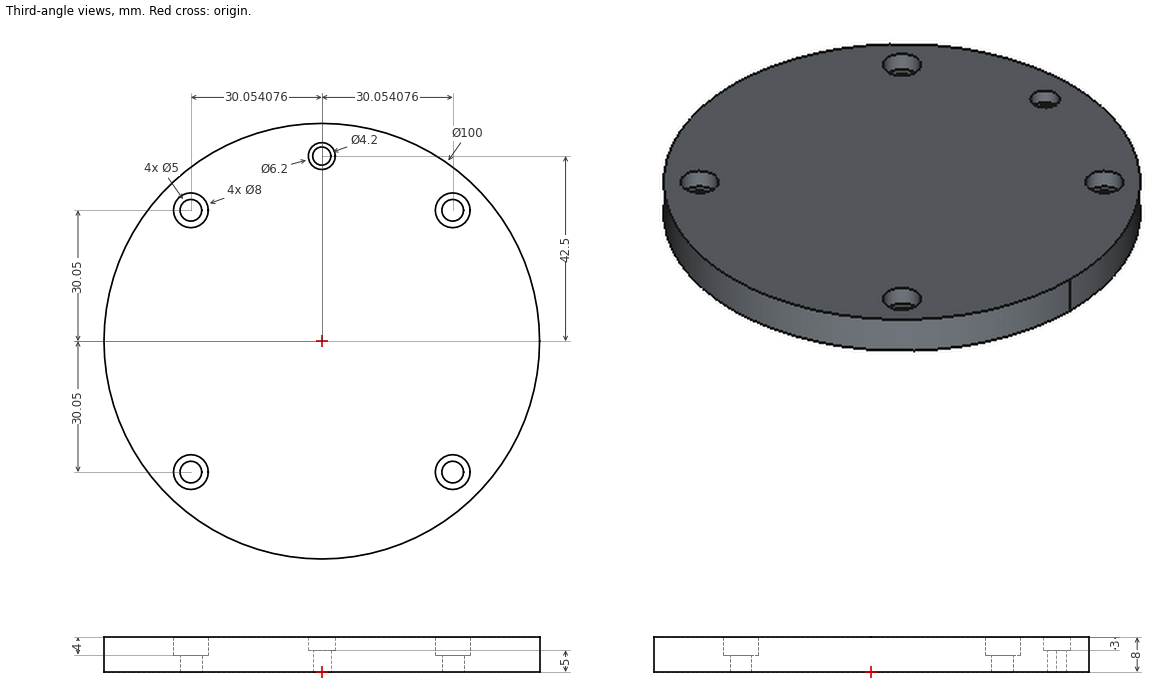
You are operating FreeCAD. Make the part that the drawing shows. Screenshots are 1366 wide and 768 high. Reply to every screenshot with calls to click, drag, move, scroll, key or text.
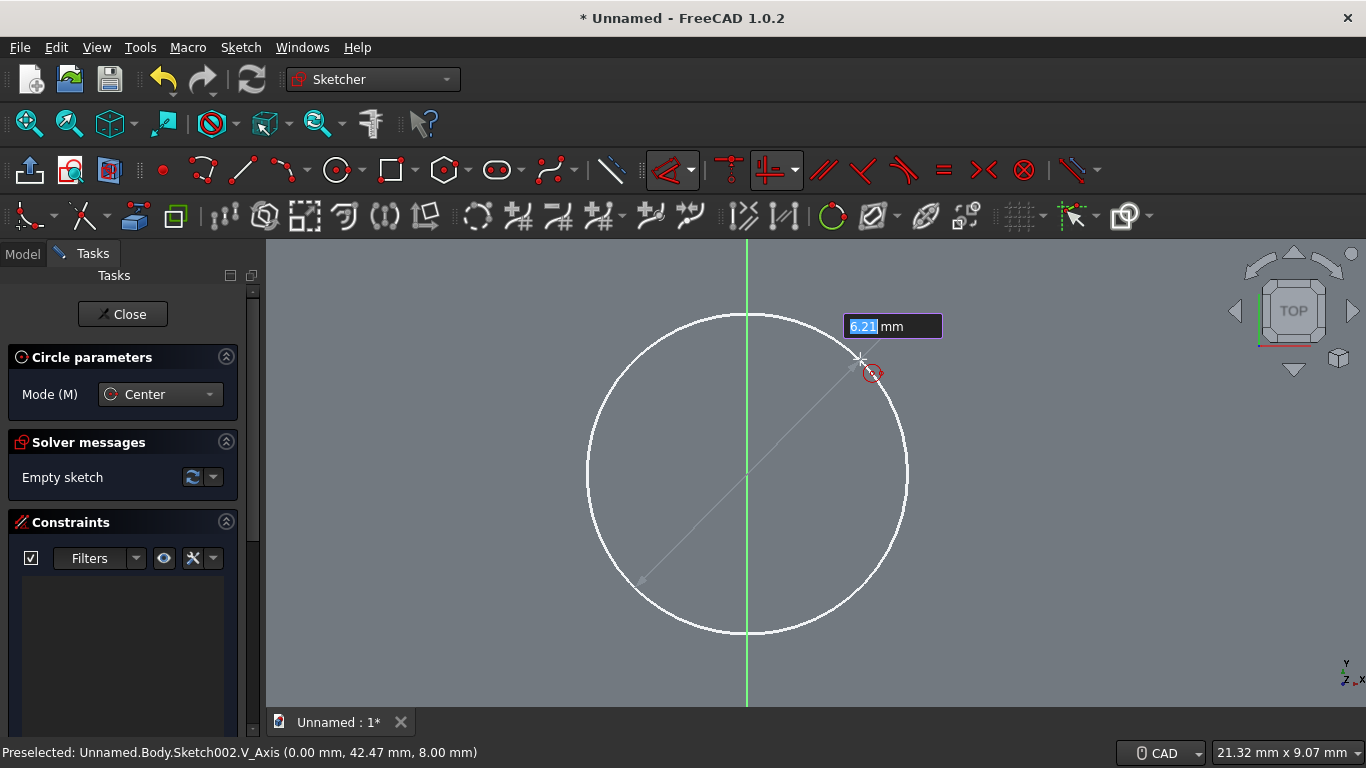
text(6.2)
key(Return)
key(Escape)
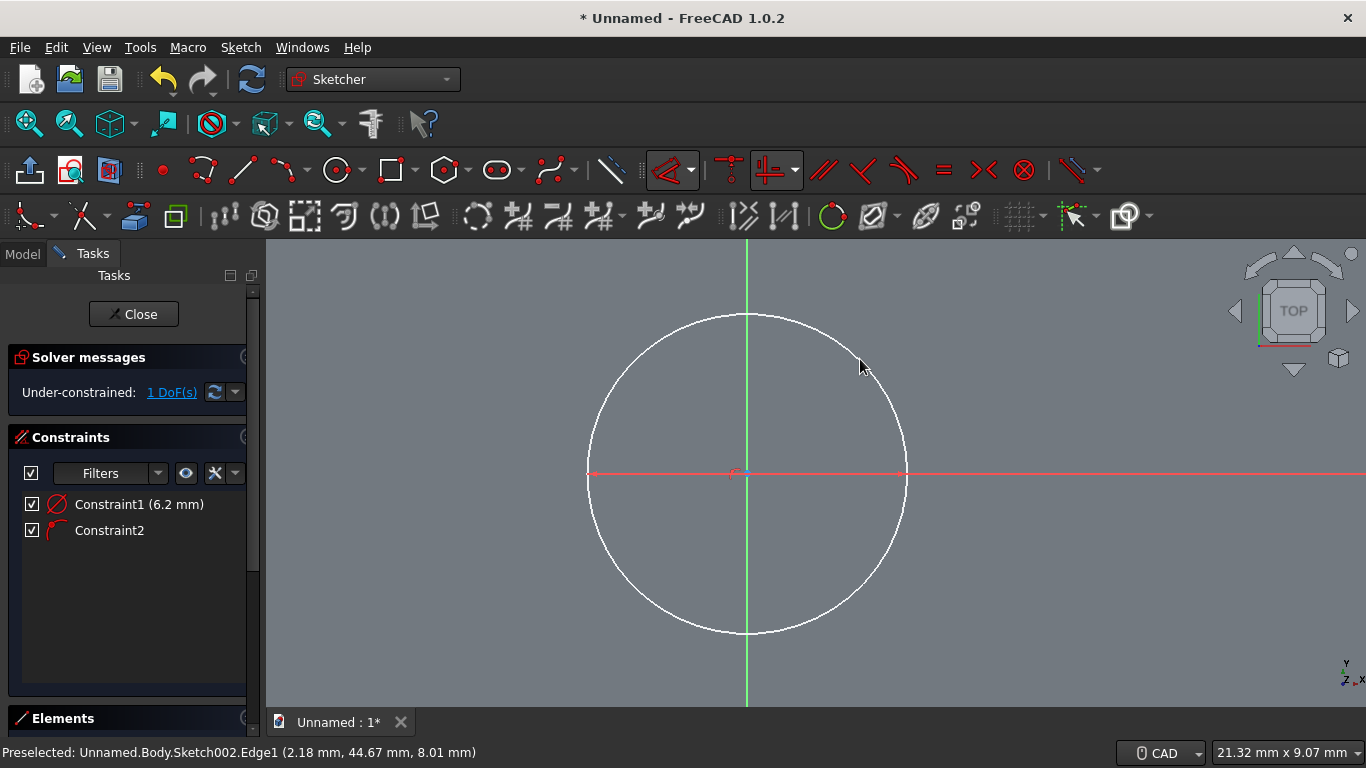
click(747, 474)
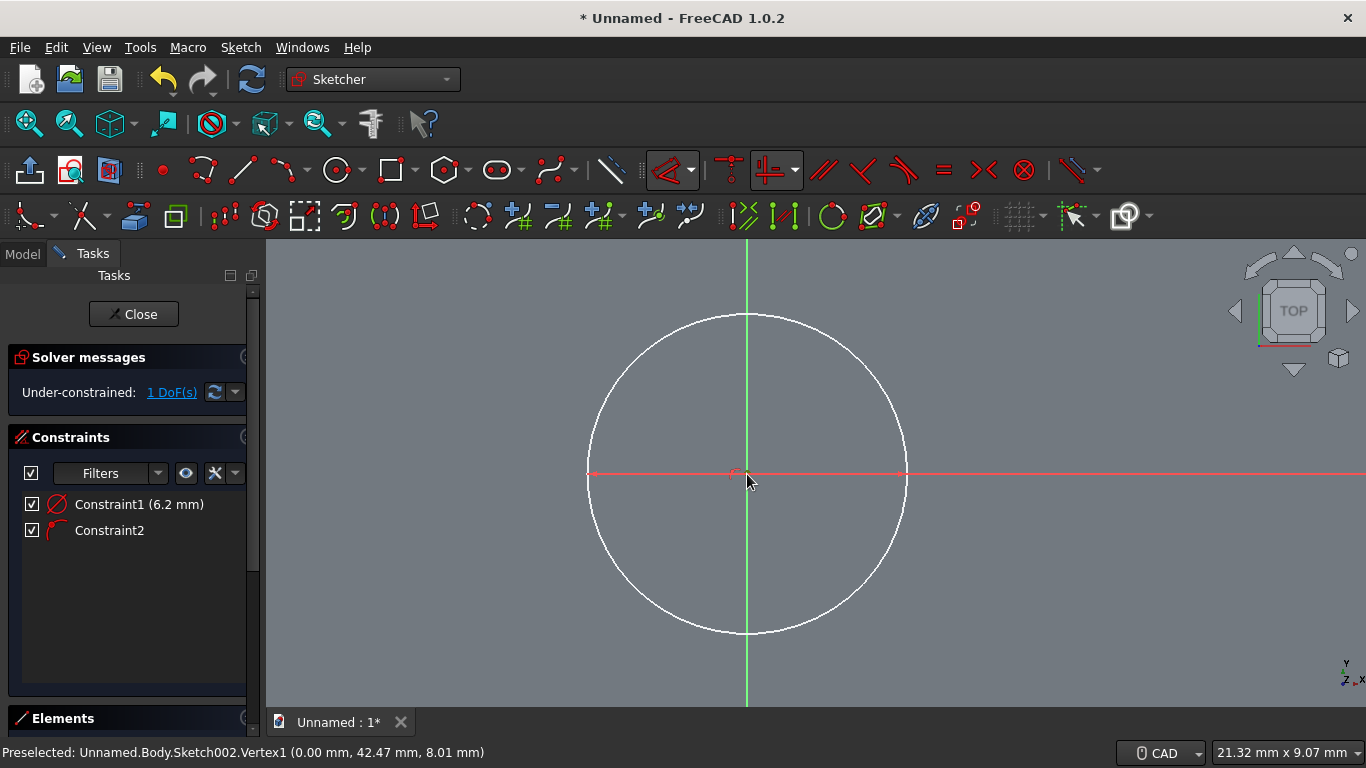
click(694, 170)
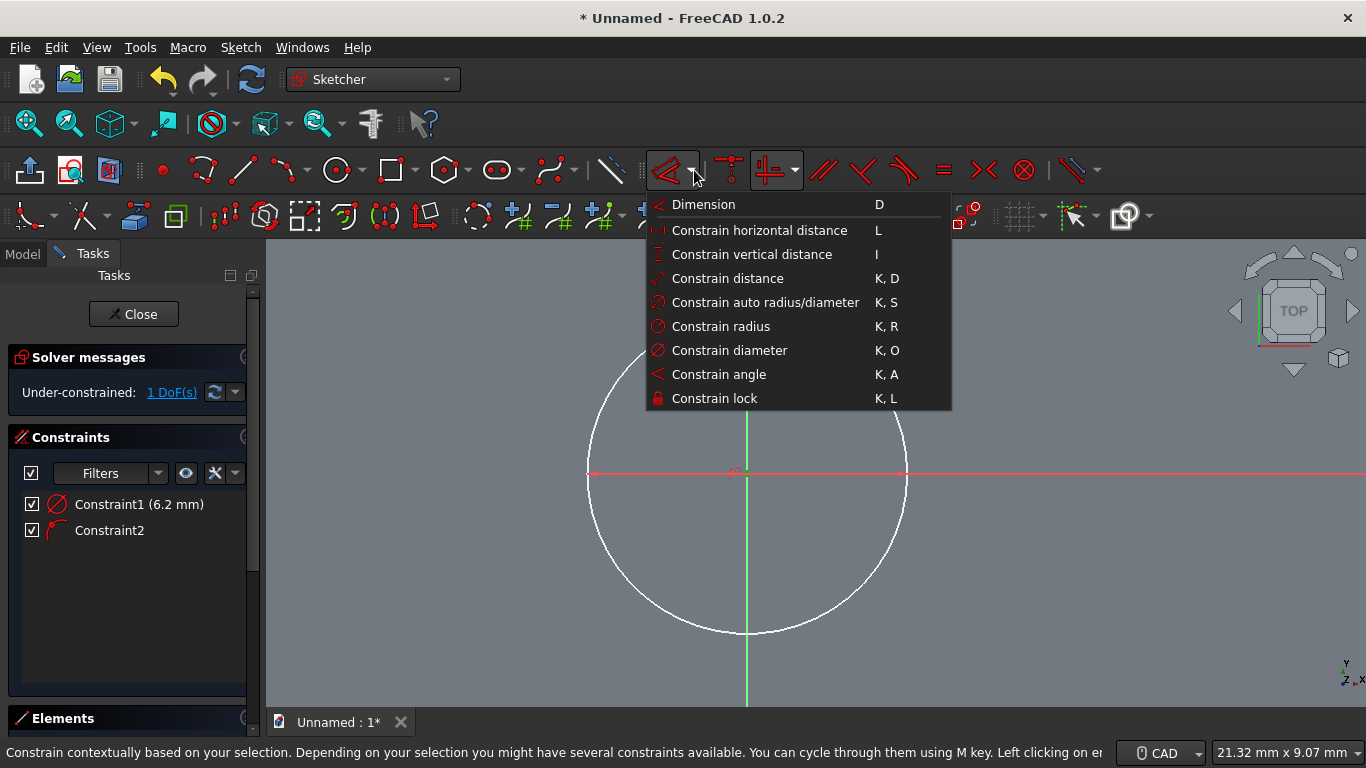
click(799, 254)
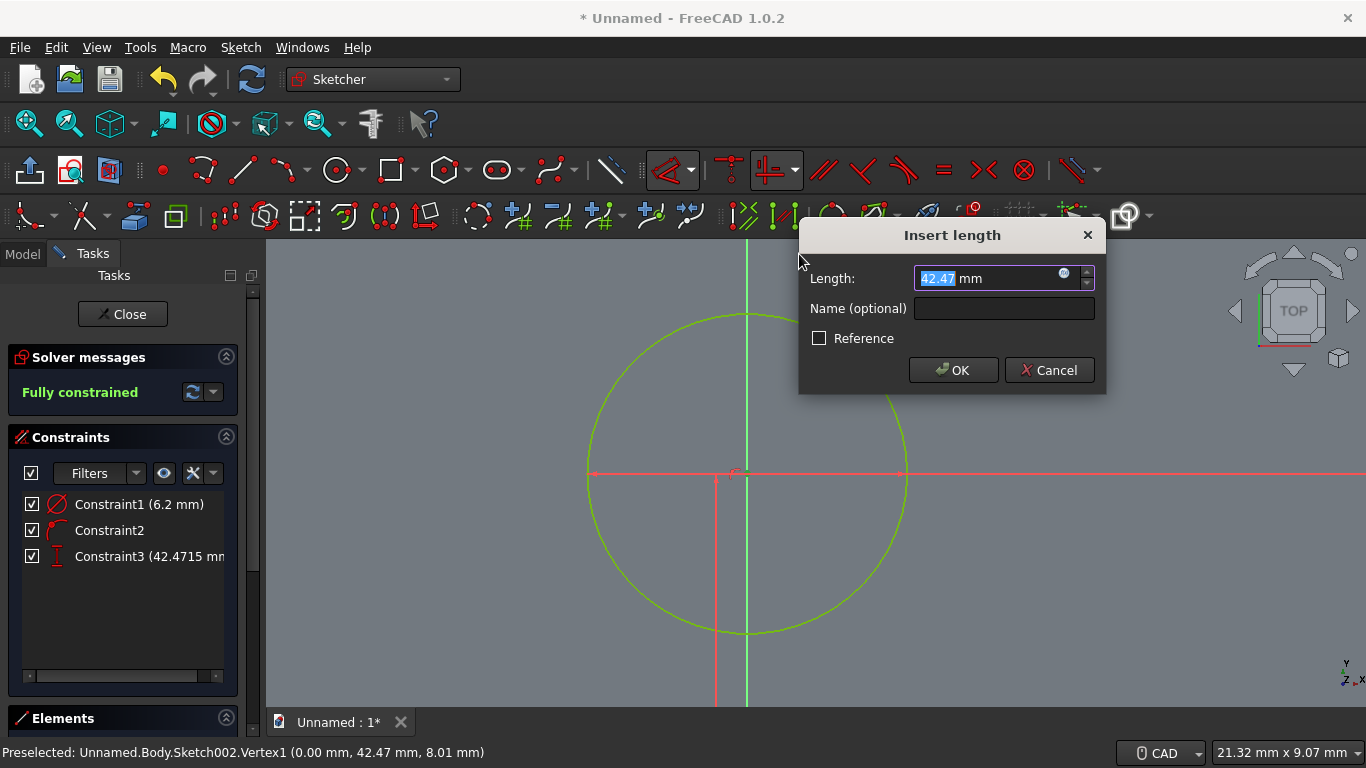
text(42.5)
key(Return)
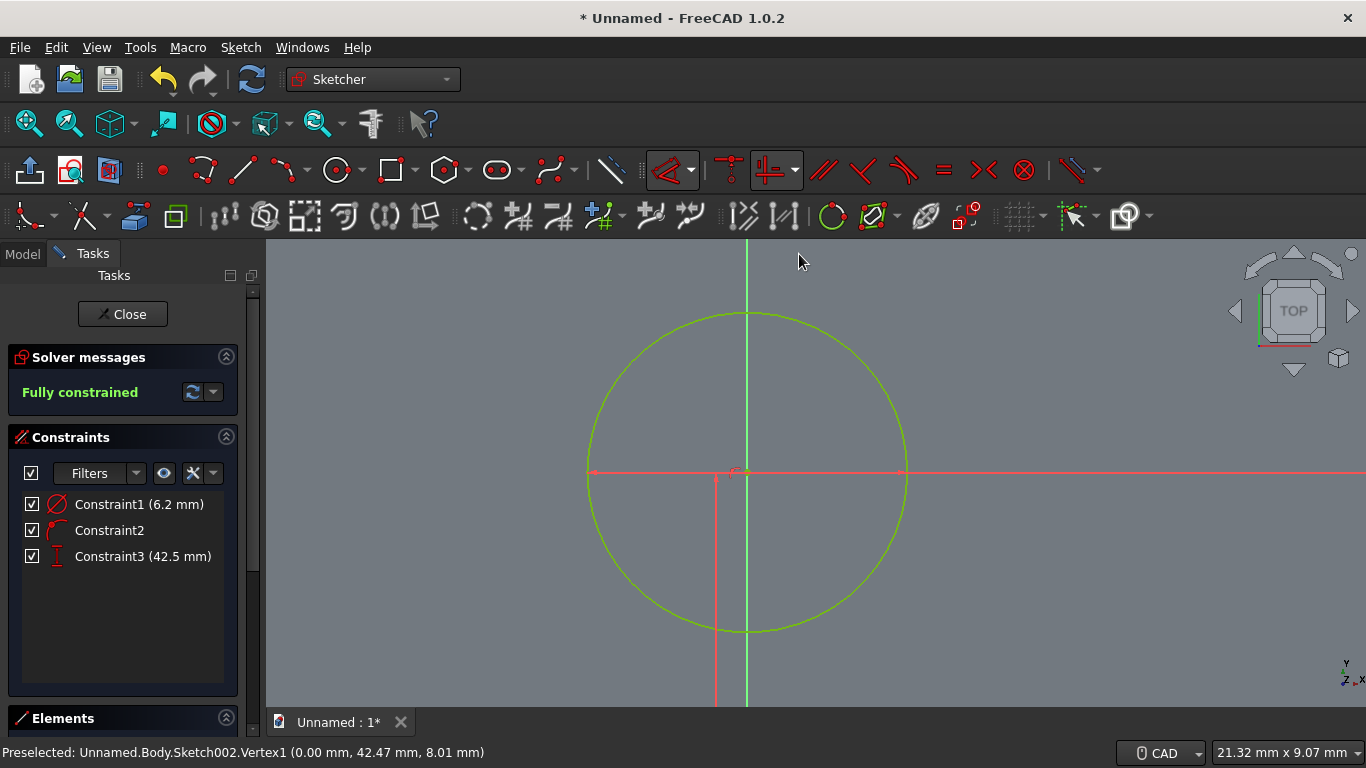
click(123, 314)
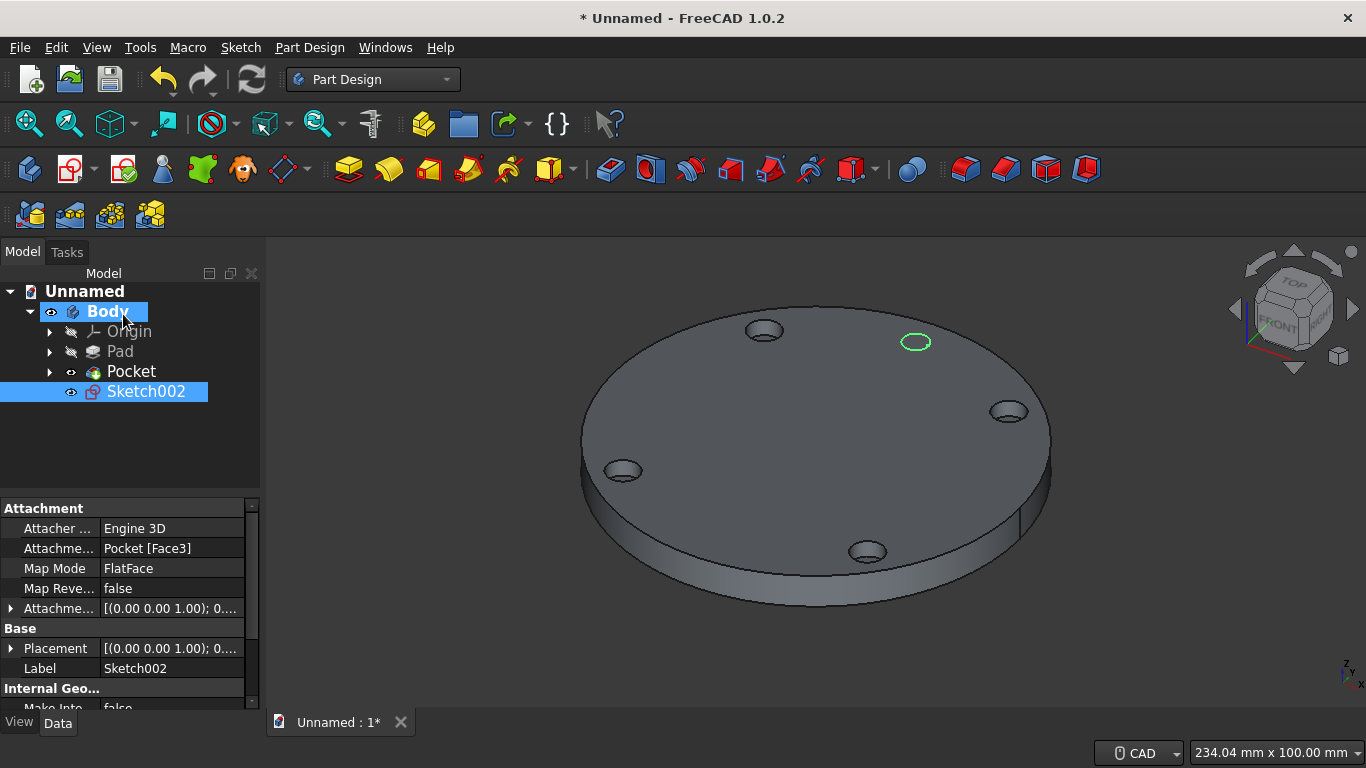
click(612, 170)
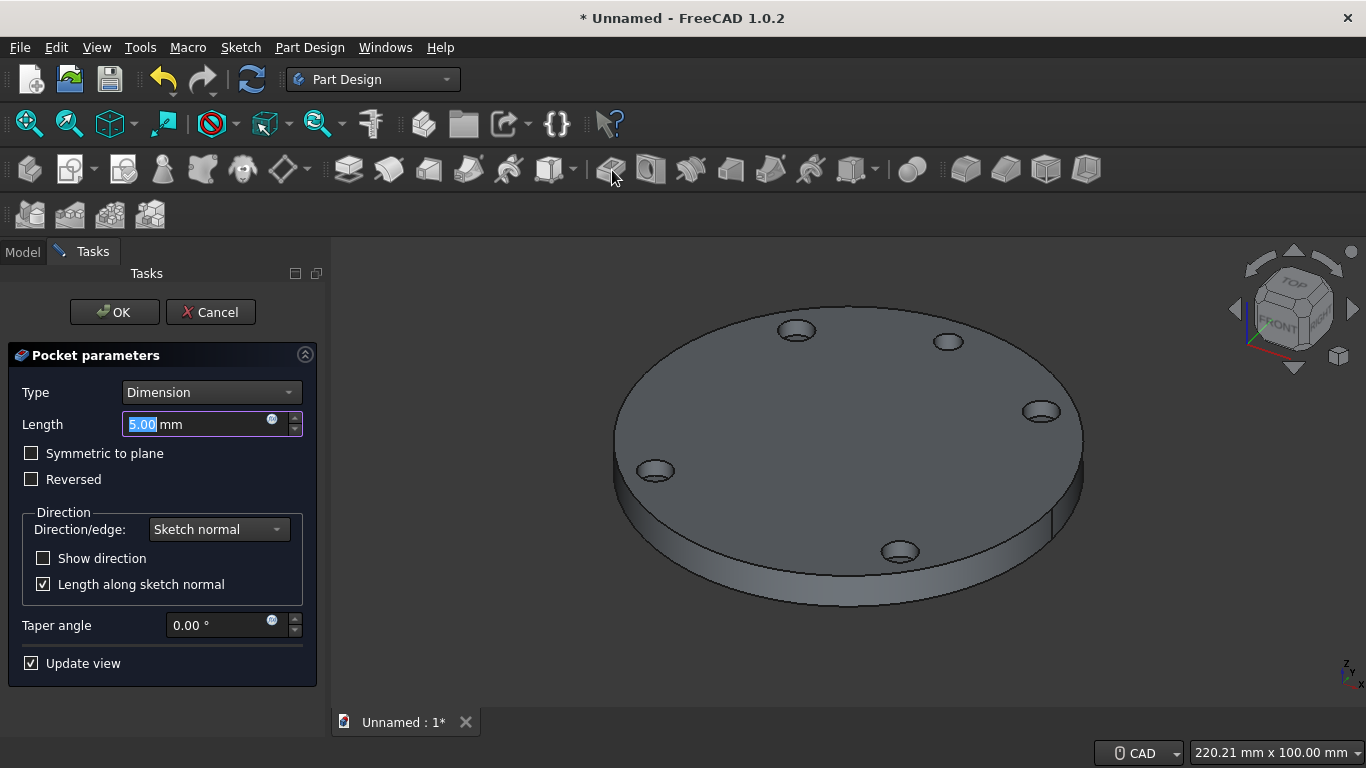
text(3)
key(Tab)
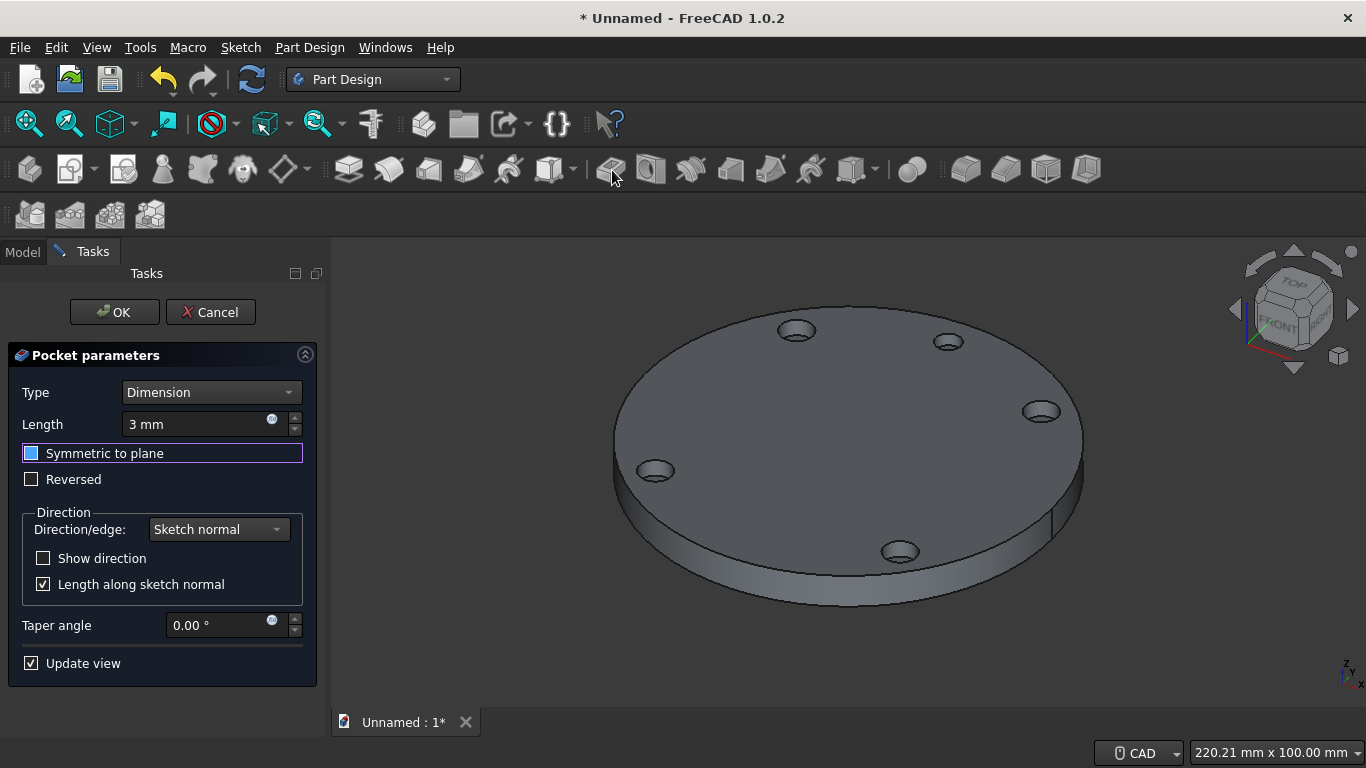
click(115, 312)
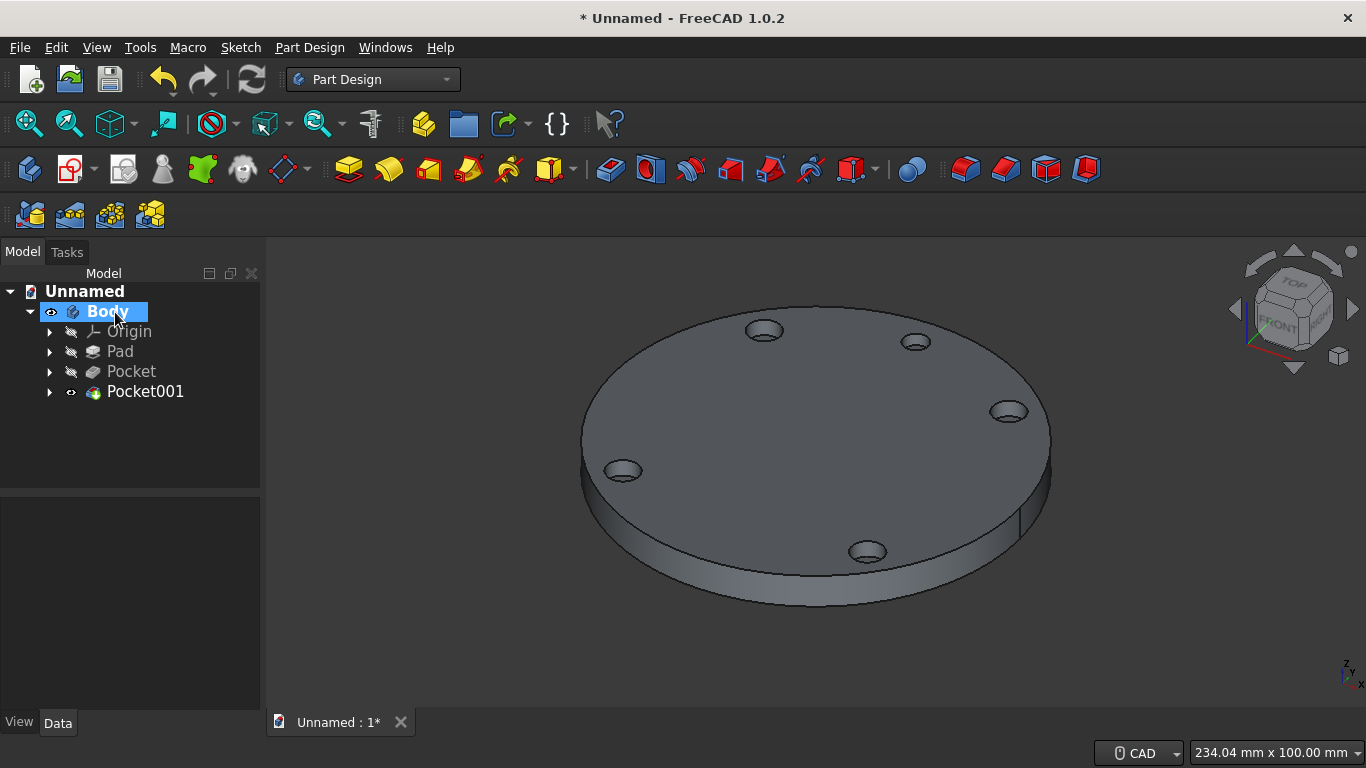
key(0)